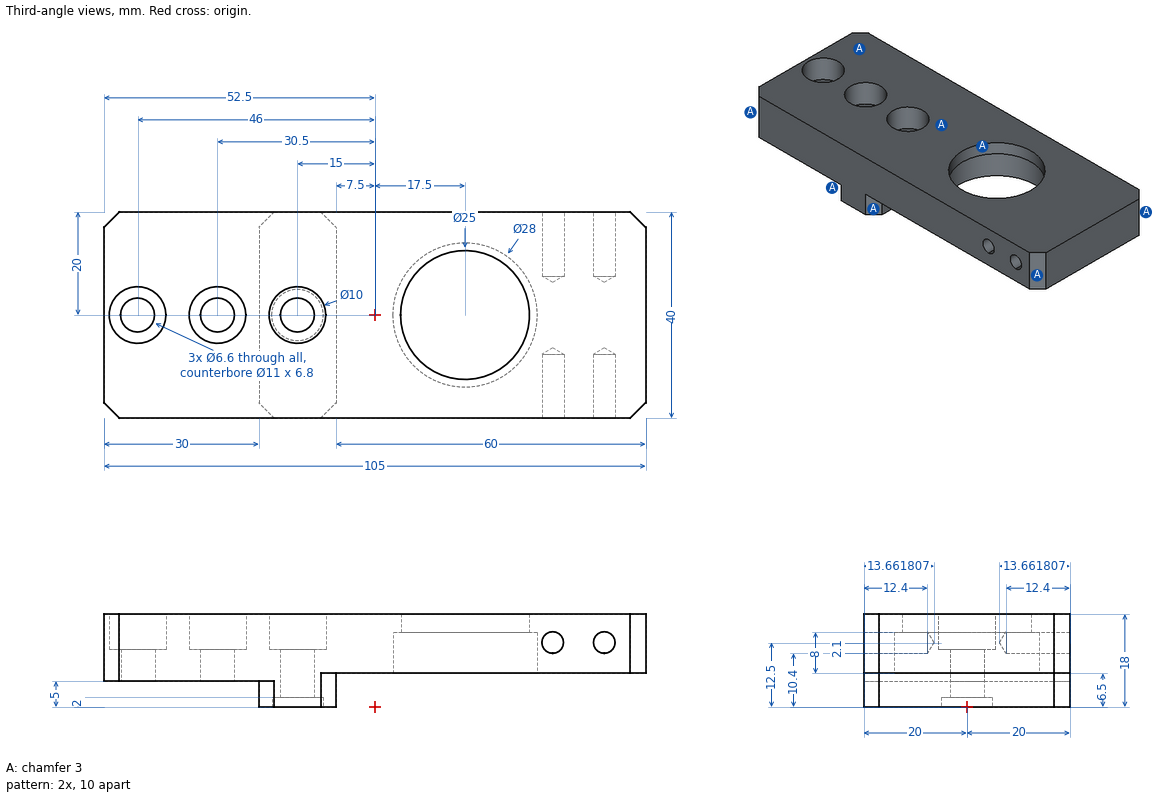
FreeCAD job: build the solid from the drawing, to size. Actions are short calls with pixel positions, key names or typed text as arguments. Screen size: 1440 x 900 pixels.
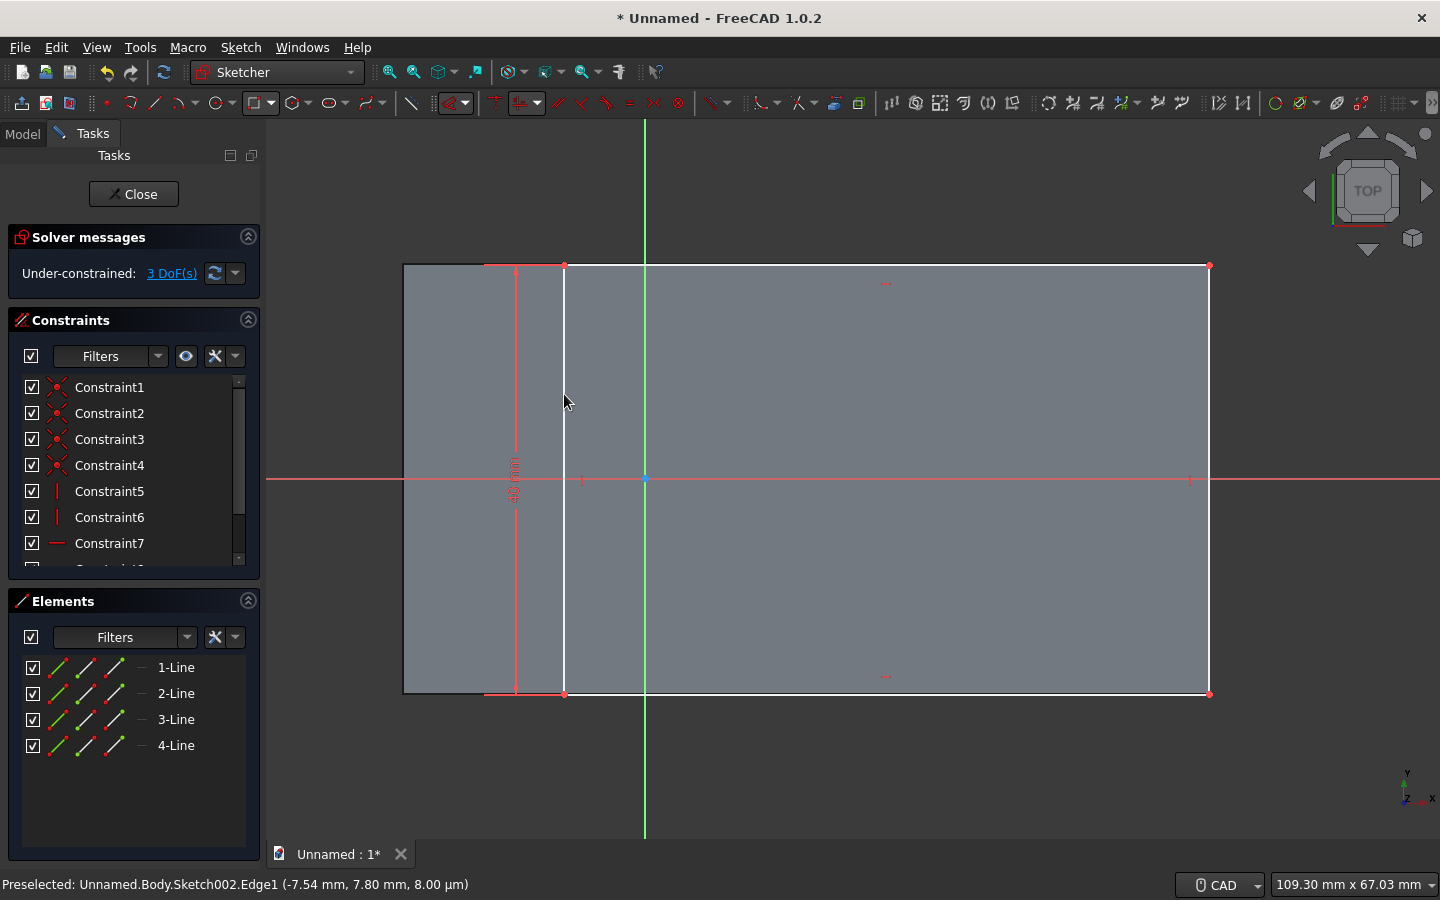
click(757, 695)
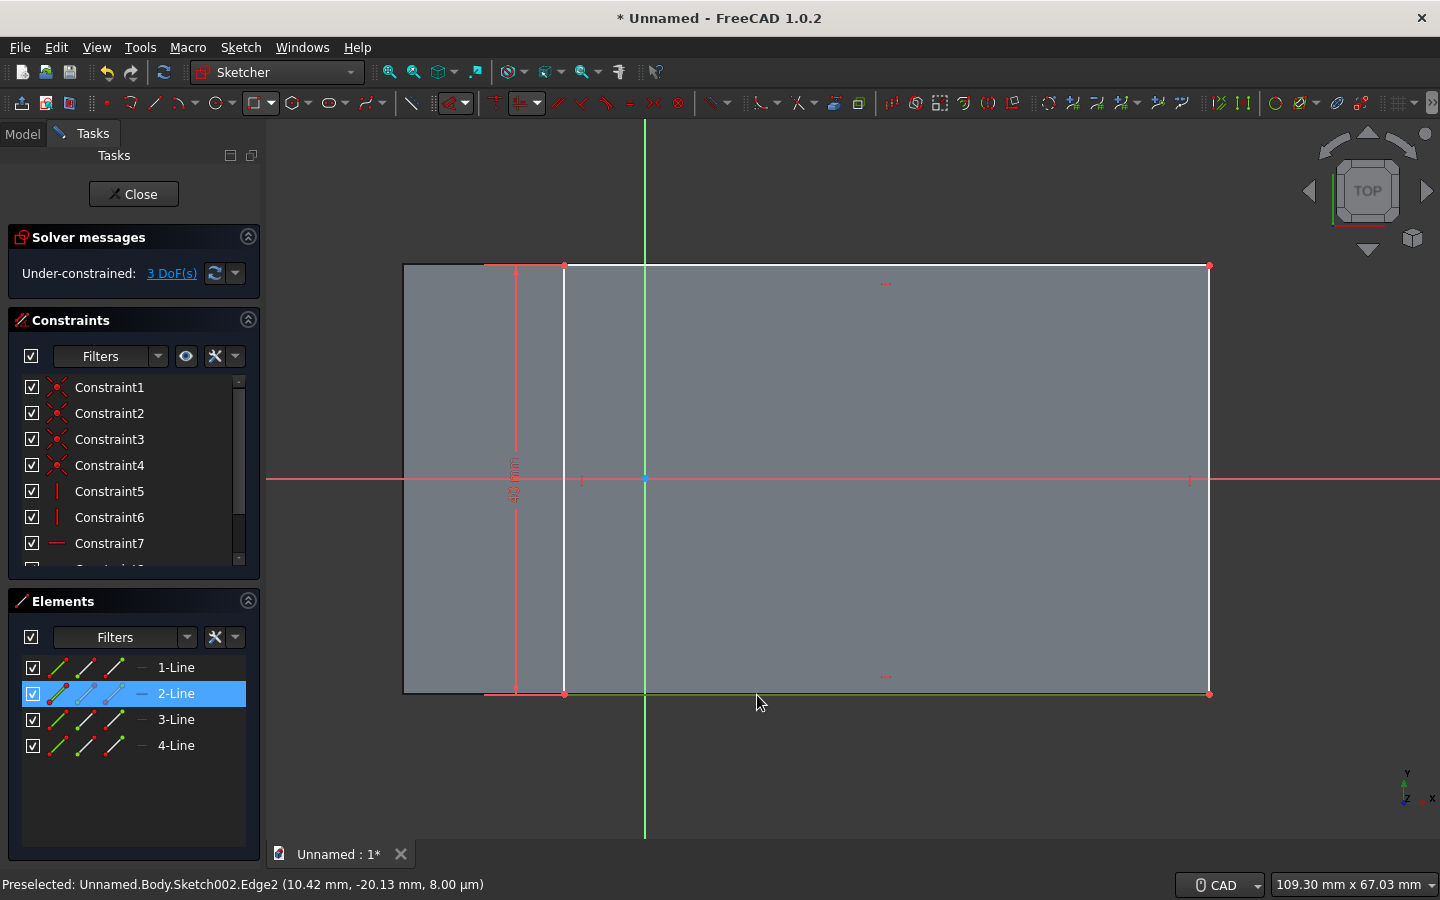
key(l)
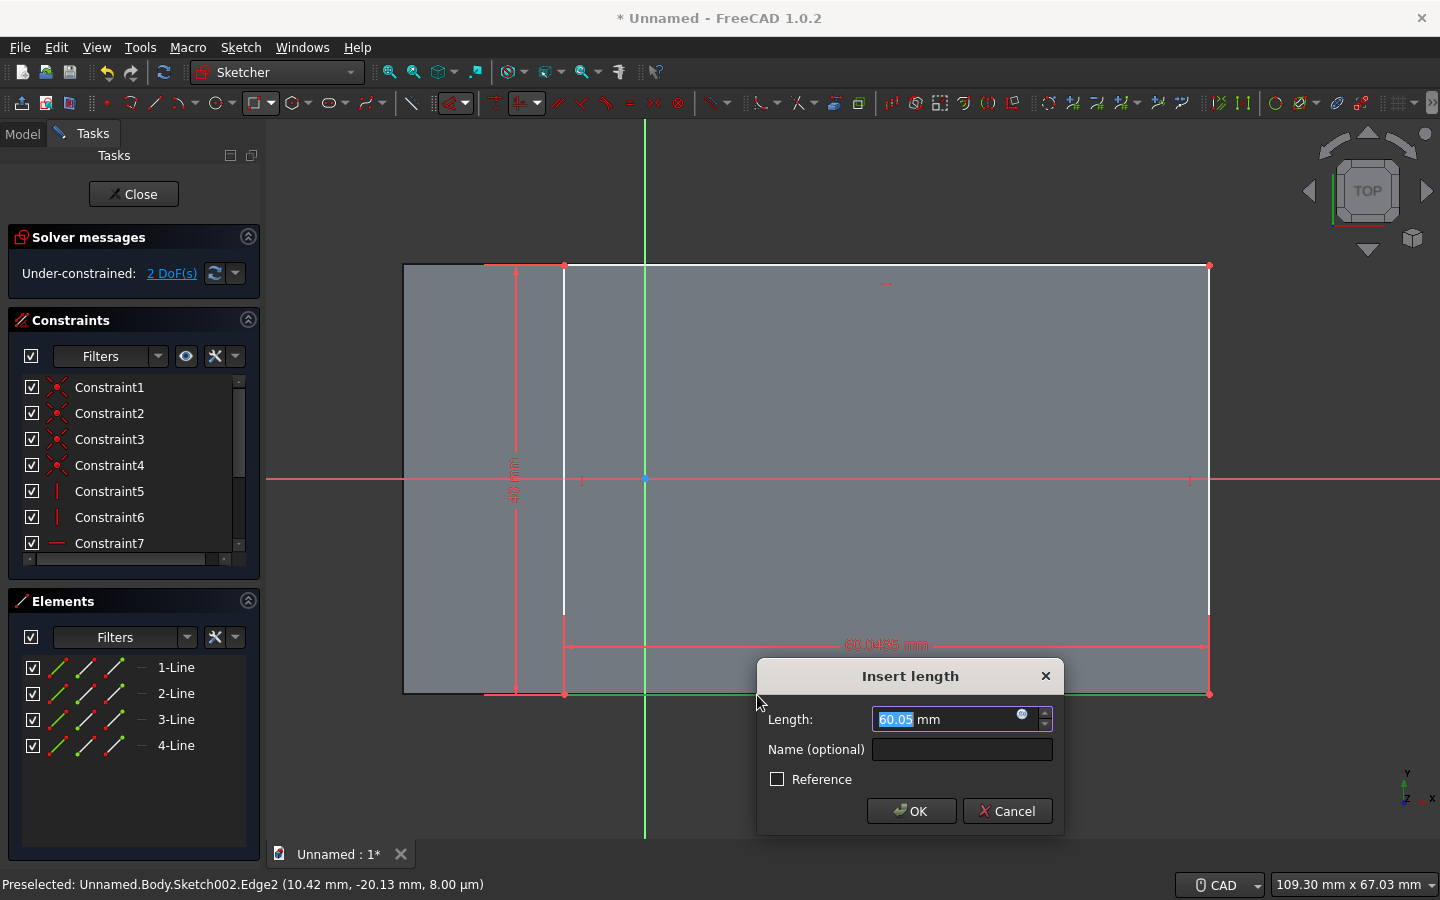
text(60)
key(Return)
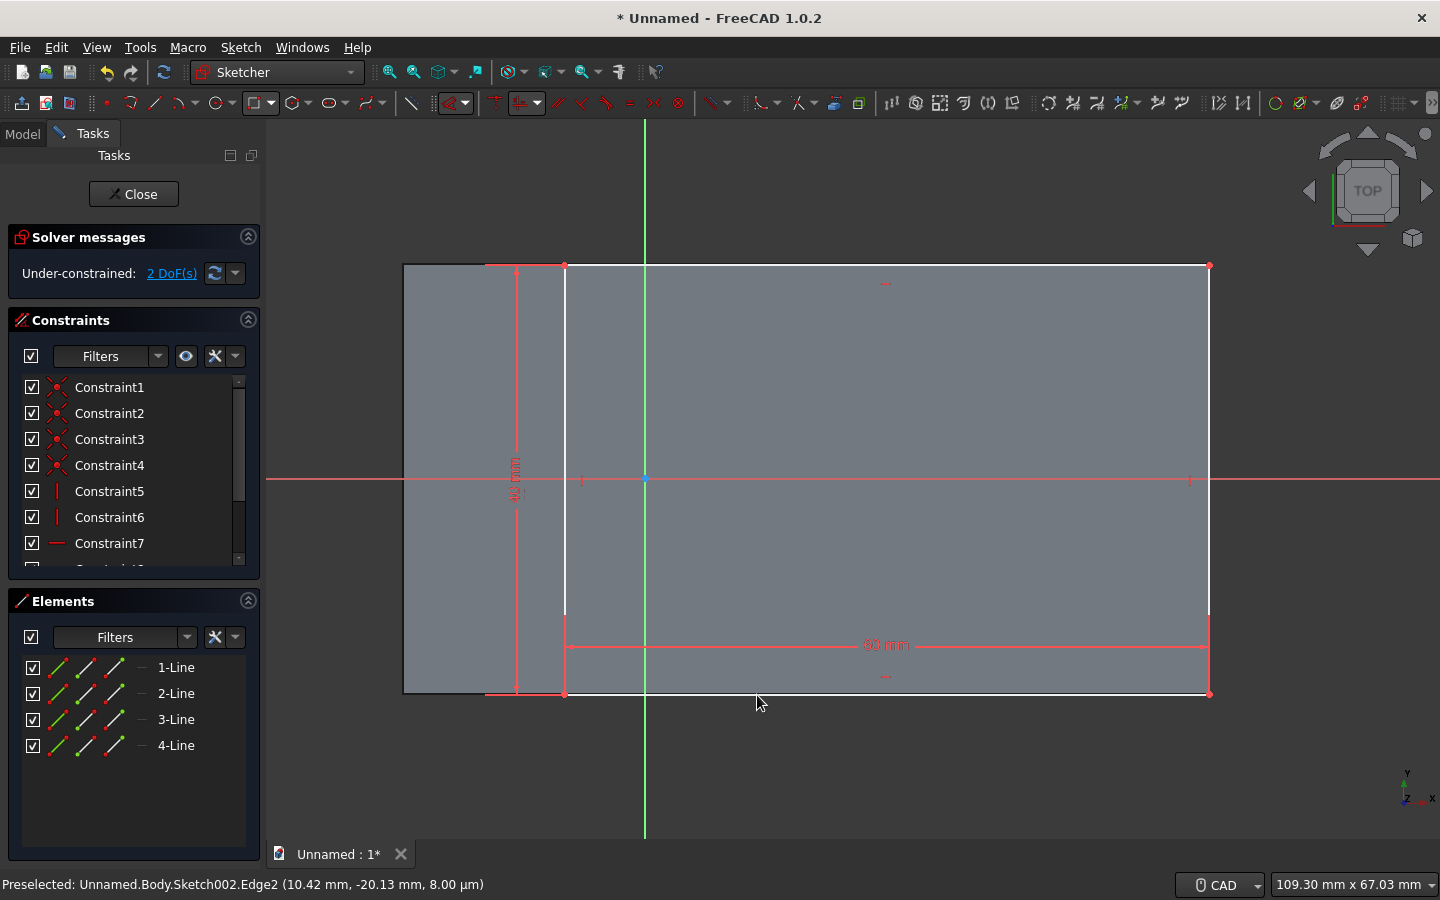
click(565, 265)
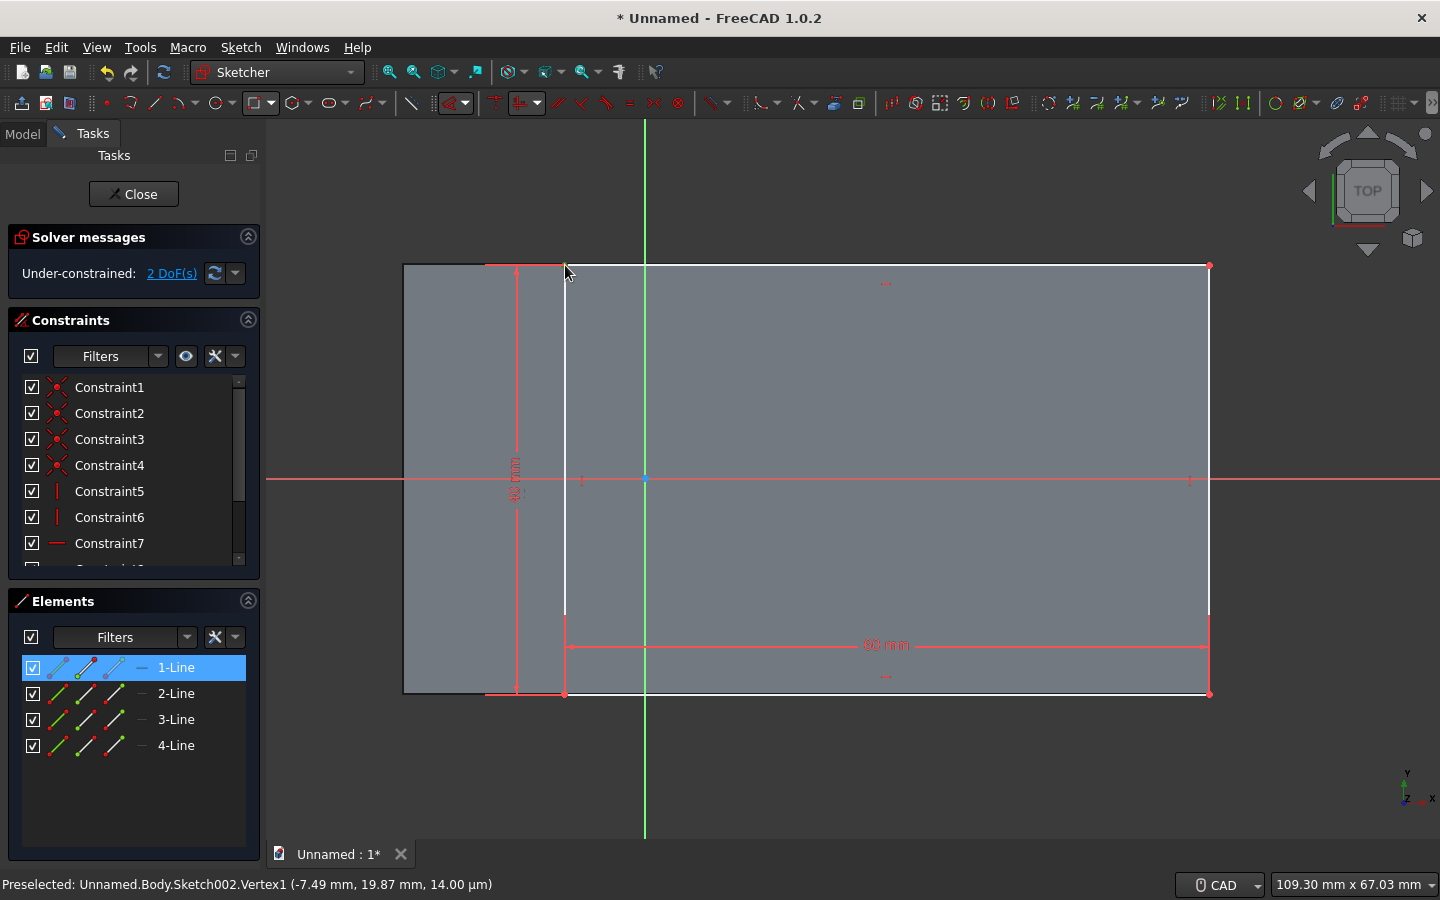
click(468, 104)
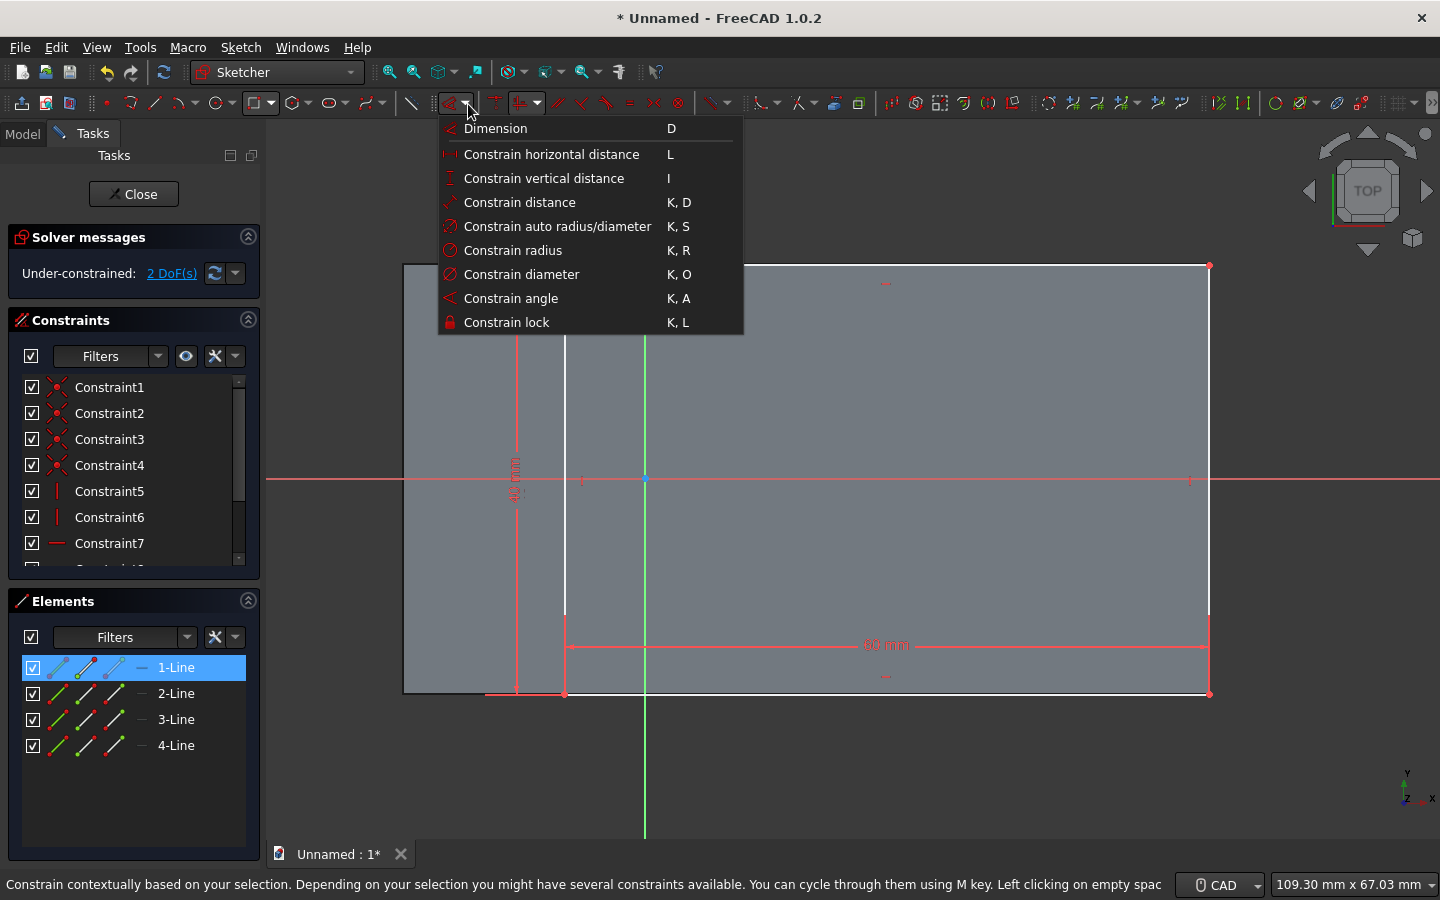
click(591, 178)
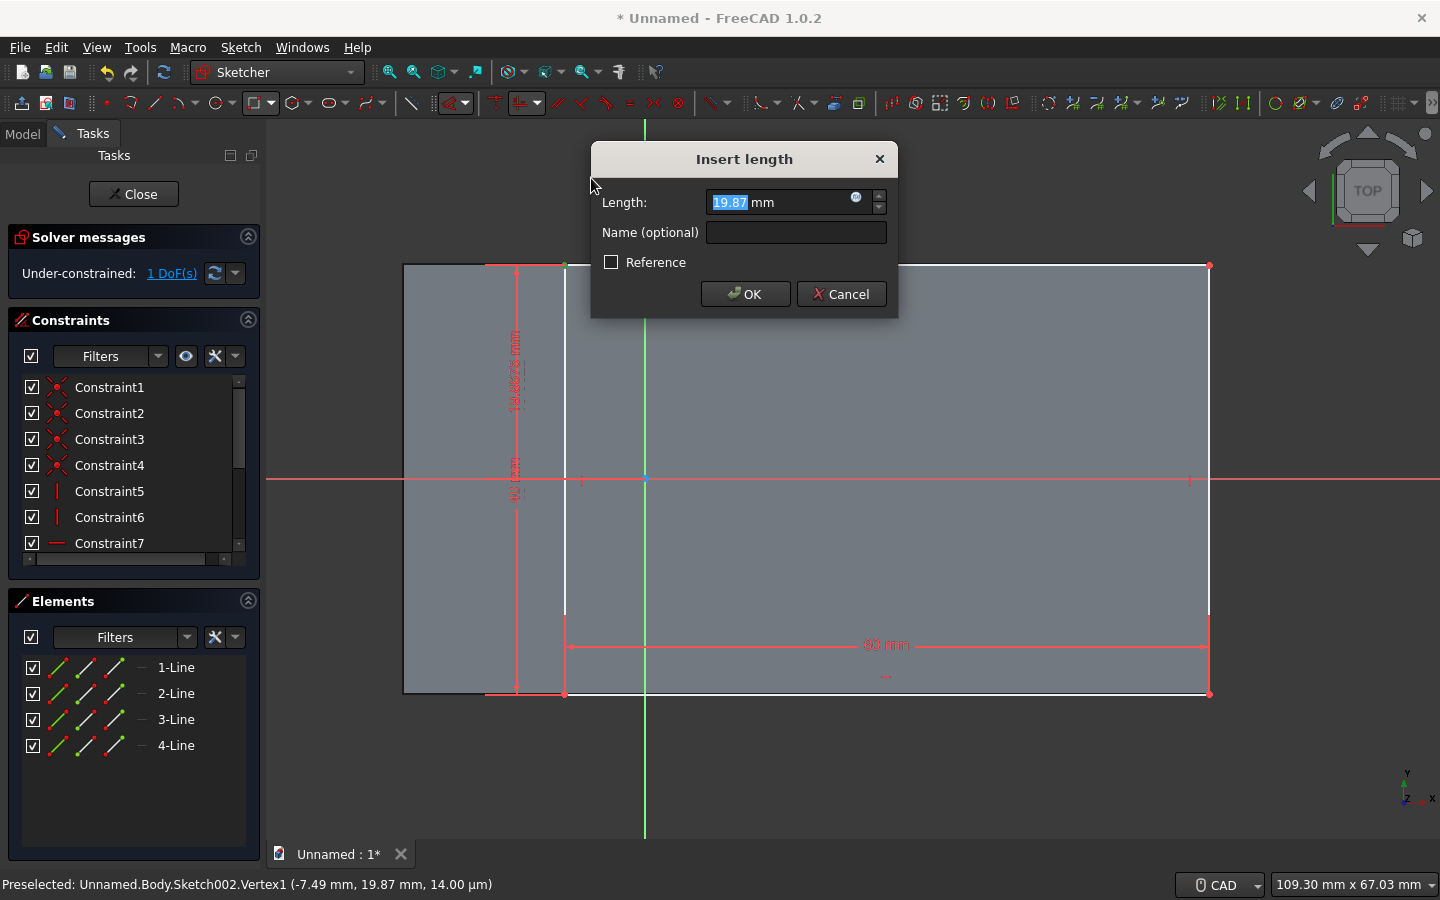
text(20)
key(Return)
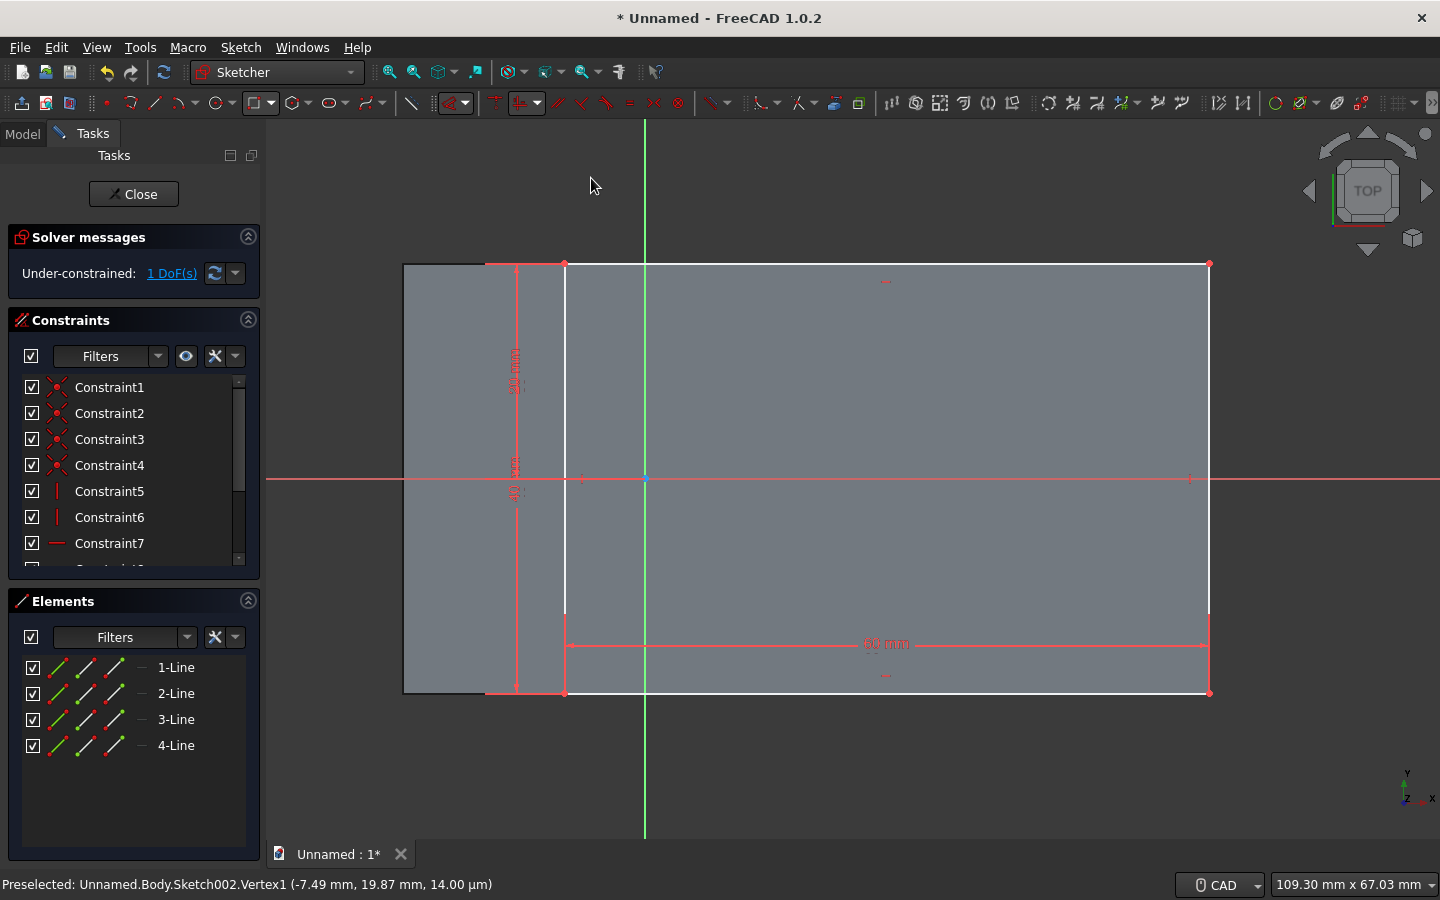
click(565, 264)